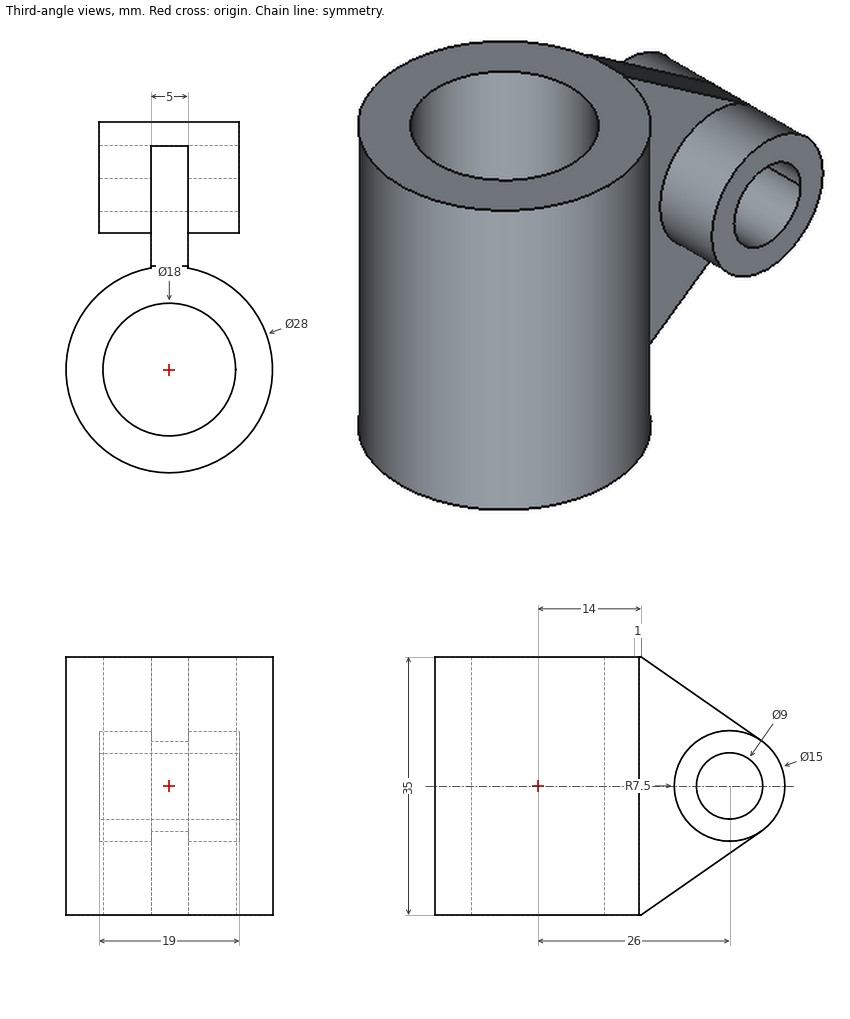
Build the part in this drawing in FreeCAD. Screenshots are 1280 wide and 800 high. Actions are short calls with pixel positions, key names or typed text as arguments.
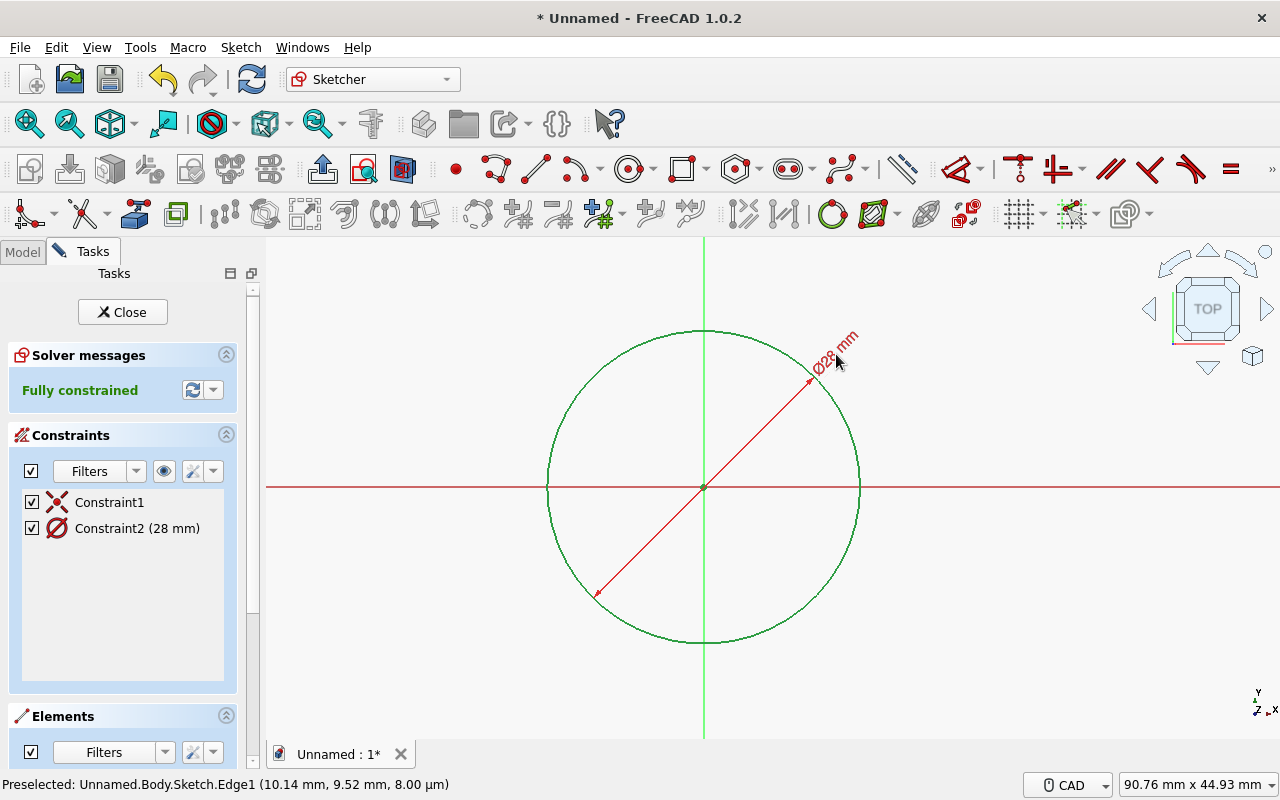
click(123, 312)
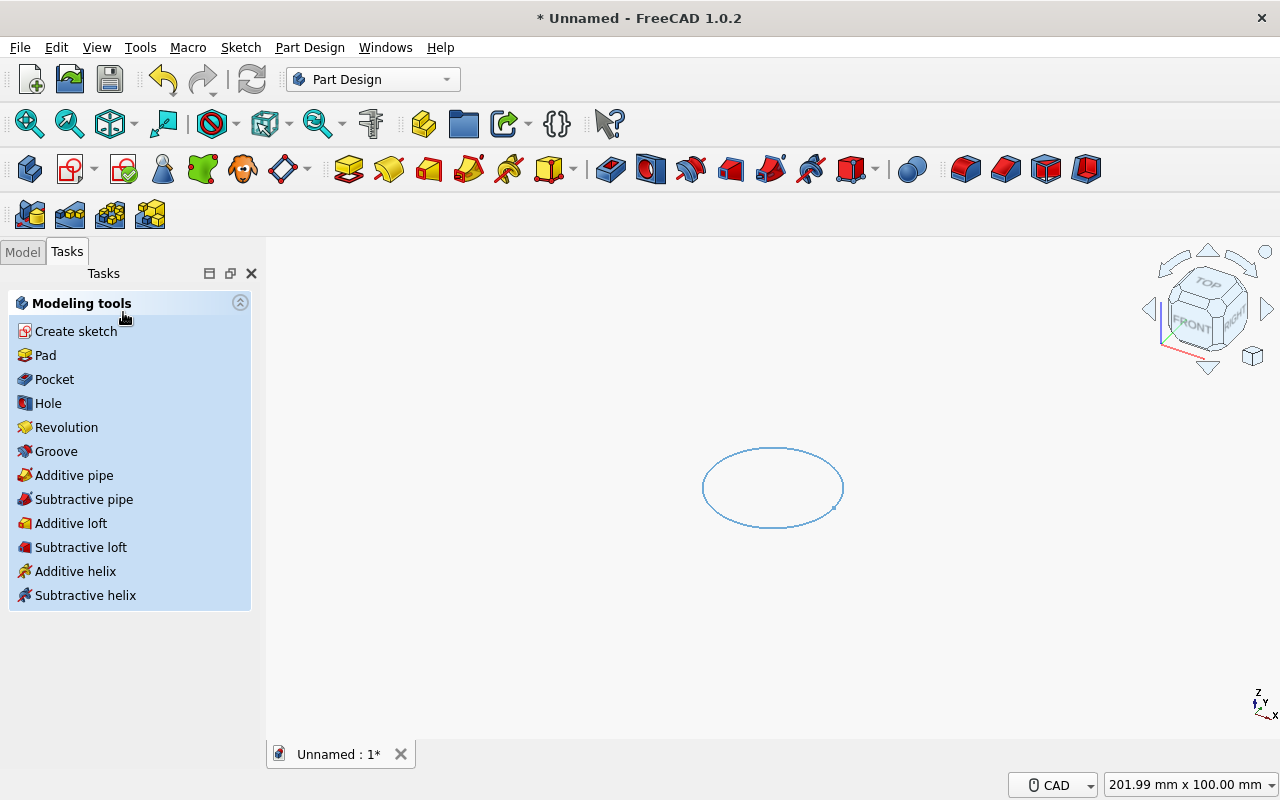
click(350, 170)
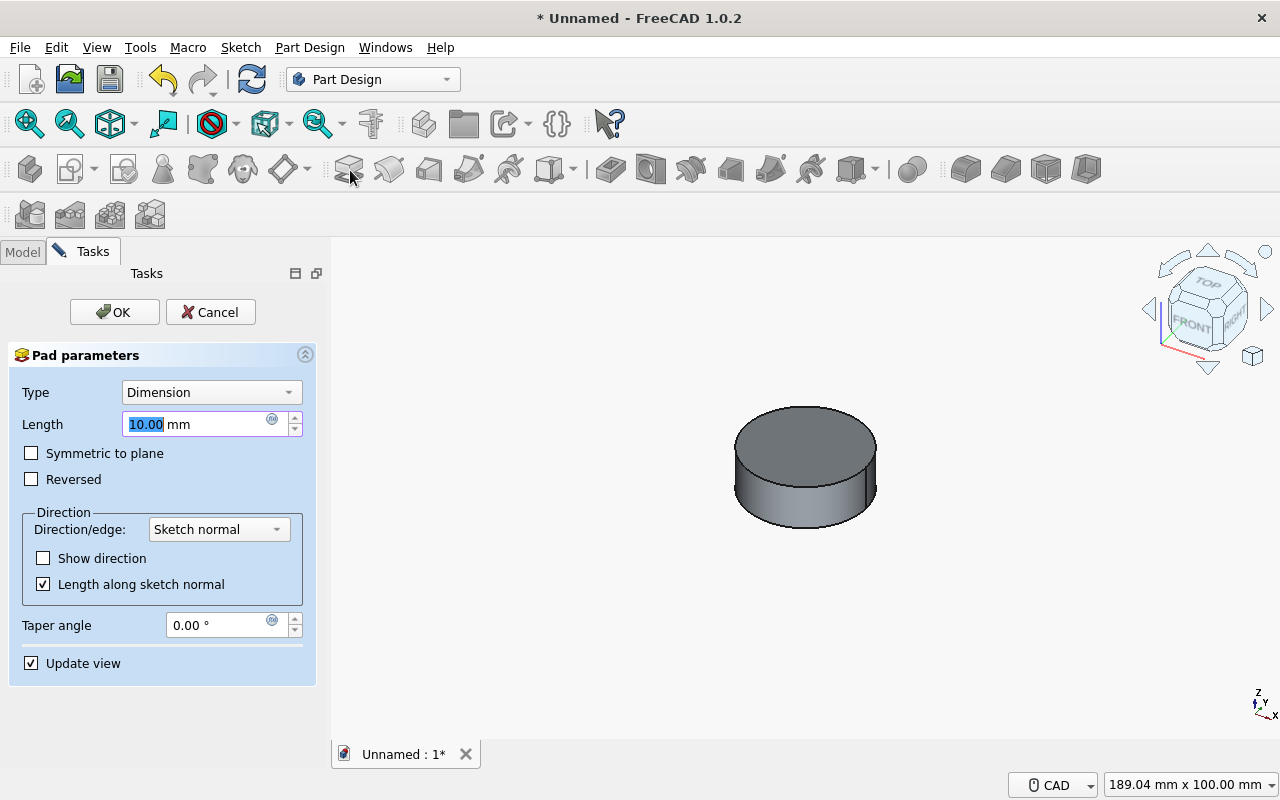
text(35)
key(Tab)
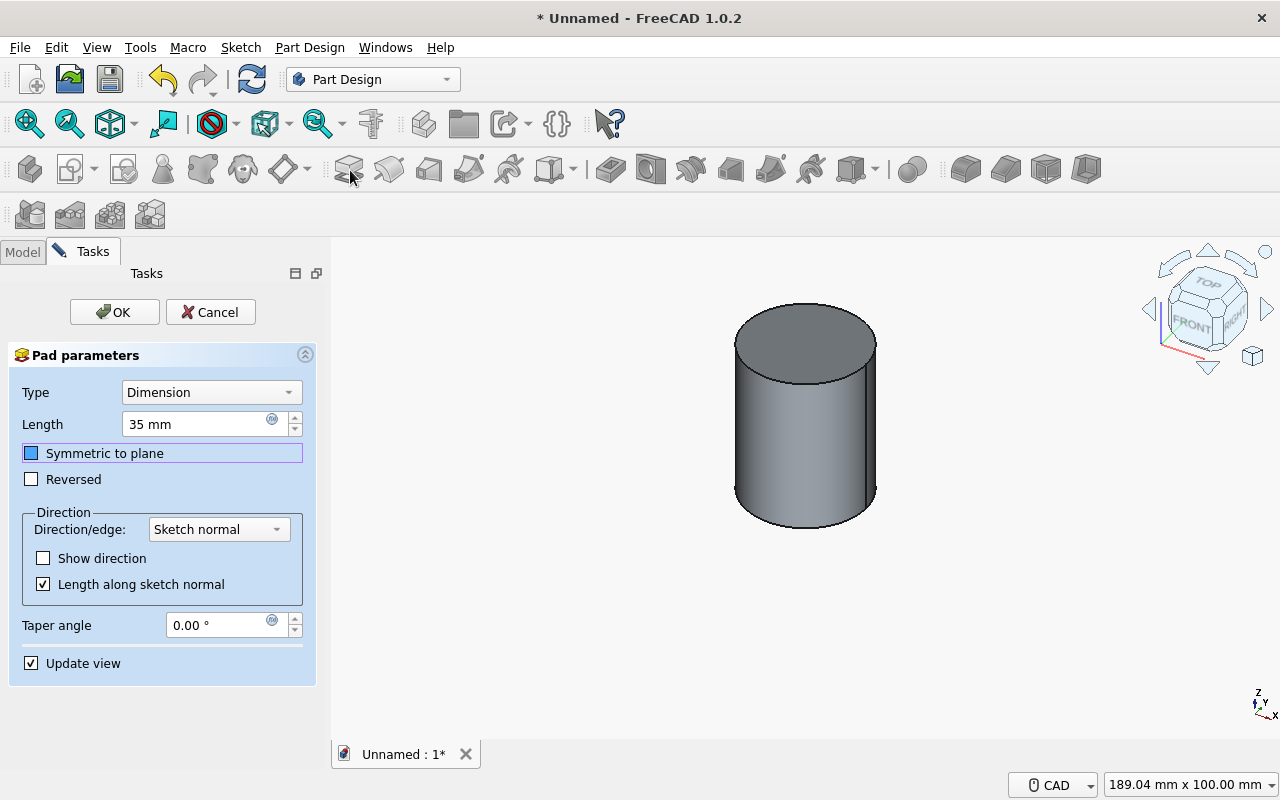
click(30, 453)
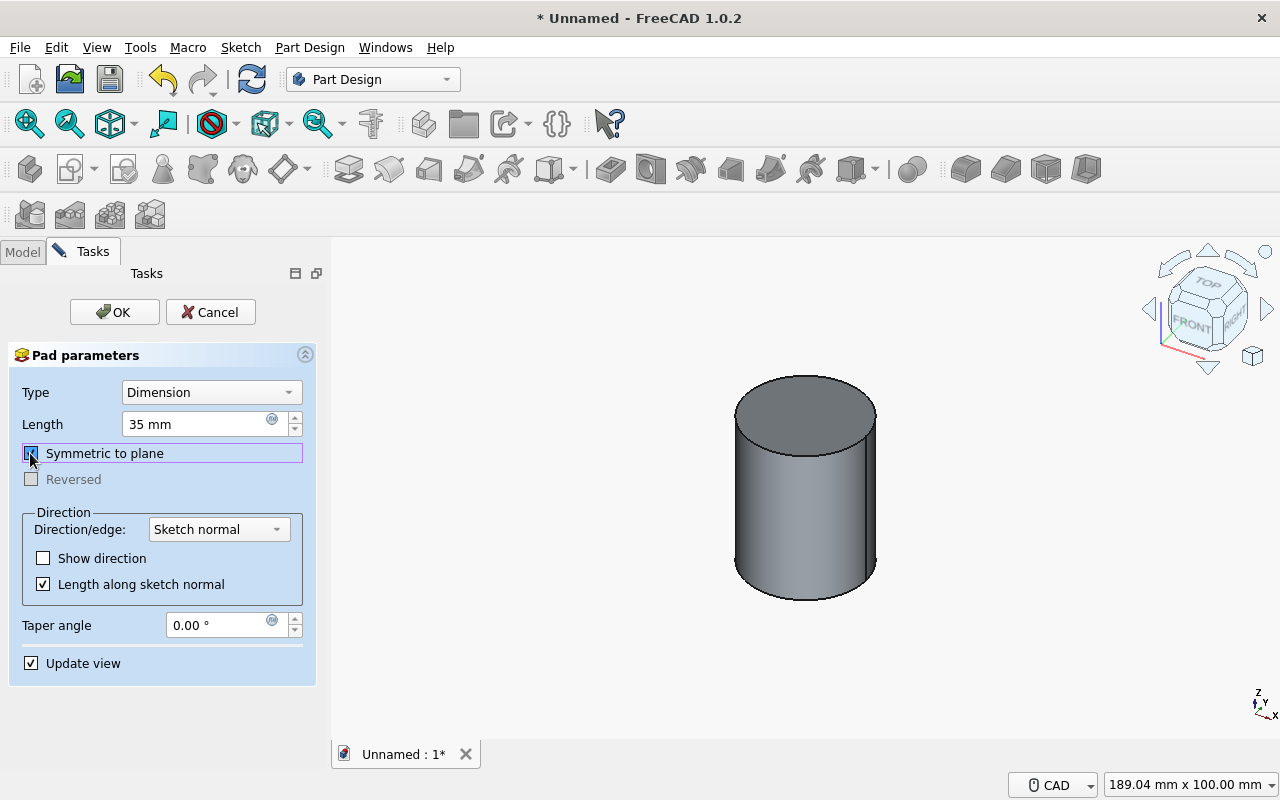
click(115, 312)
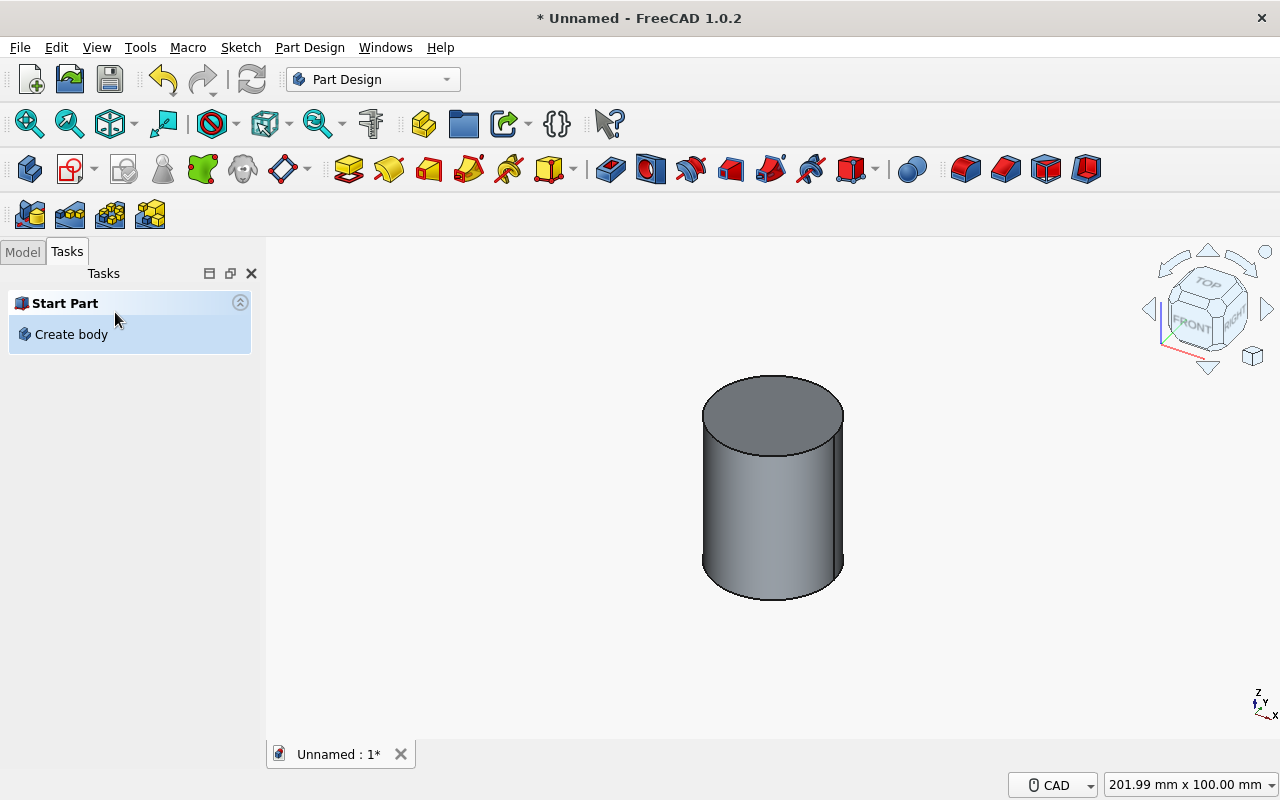
click(773, 415)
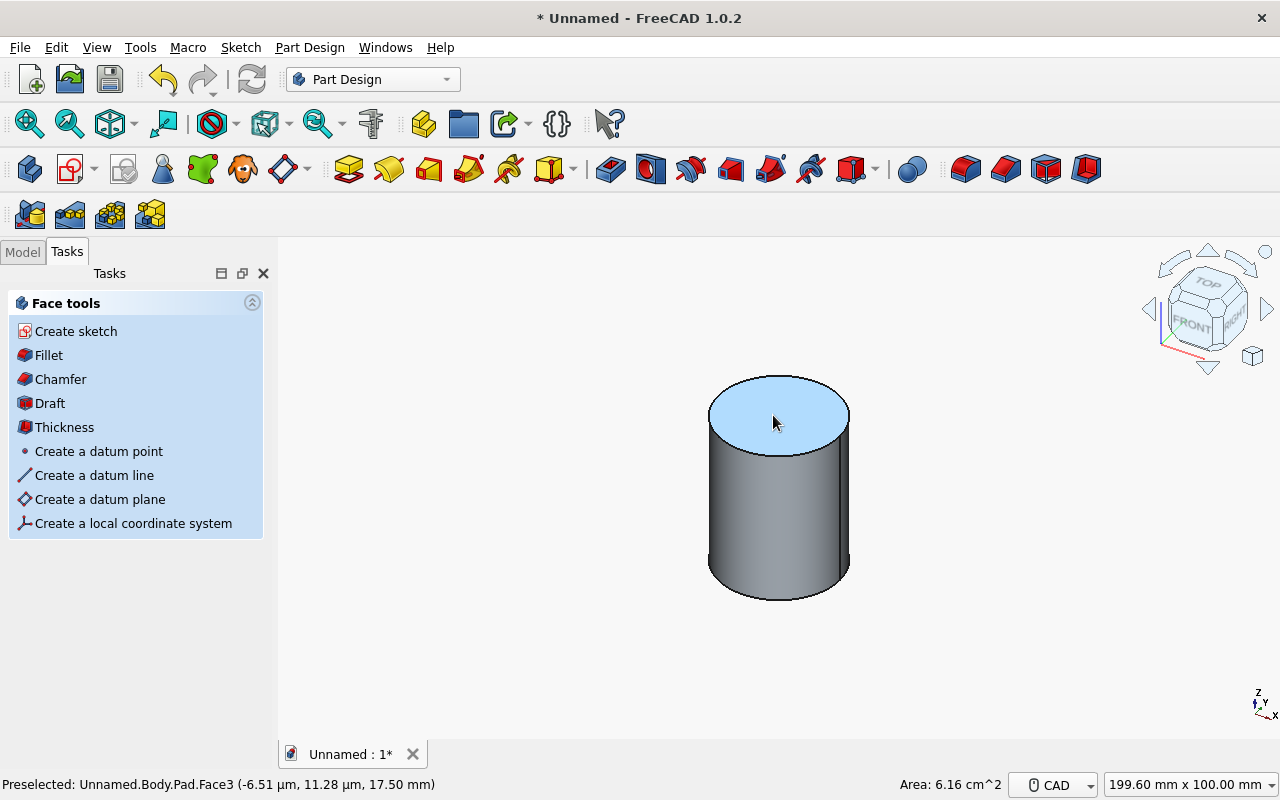
click(70, 170)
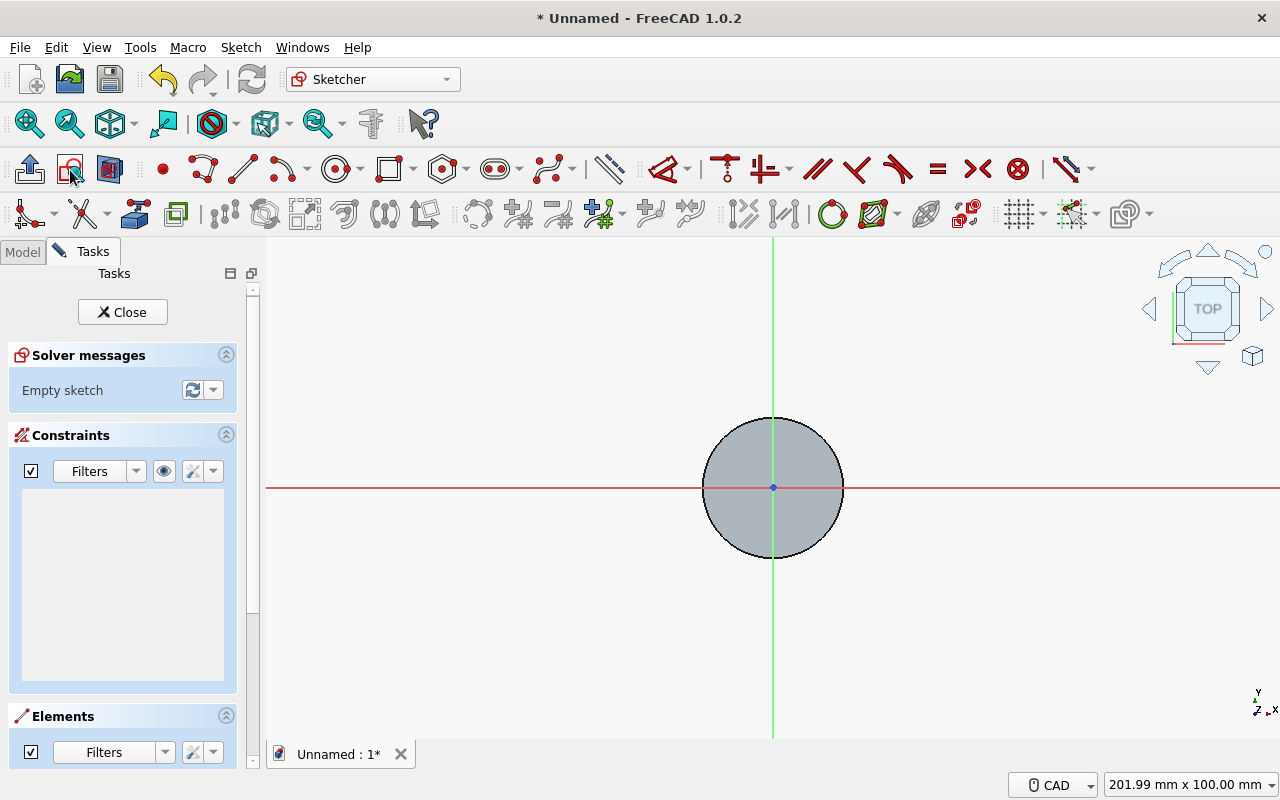
scroll(803, 488, up, 6)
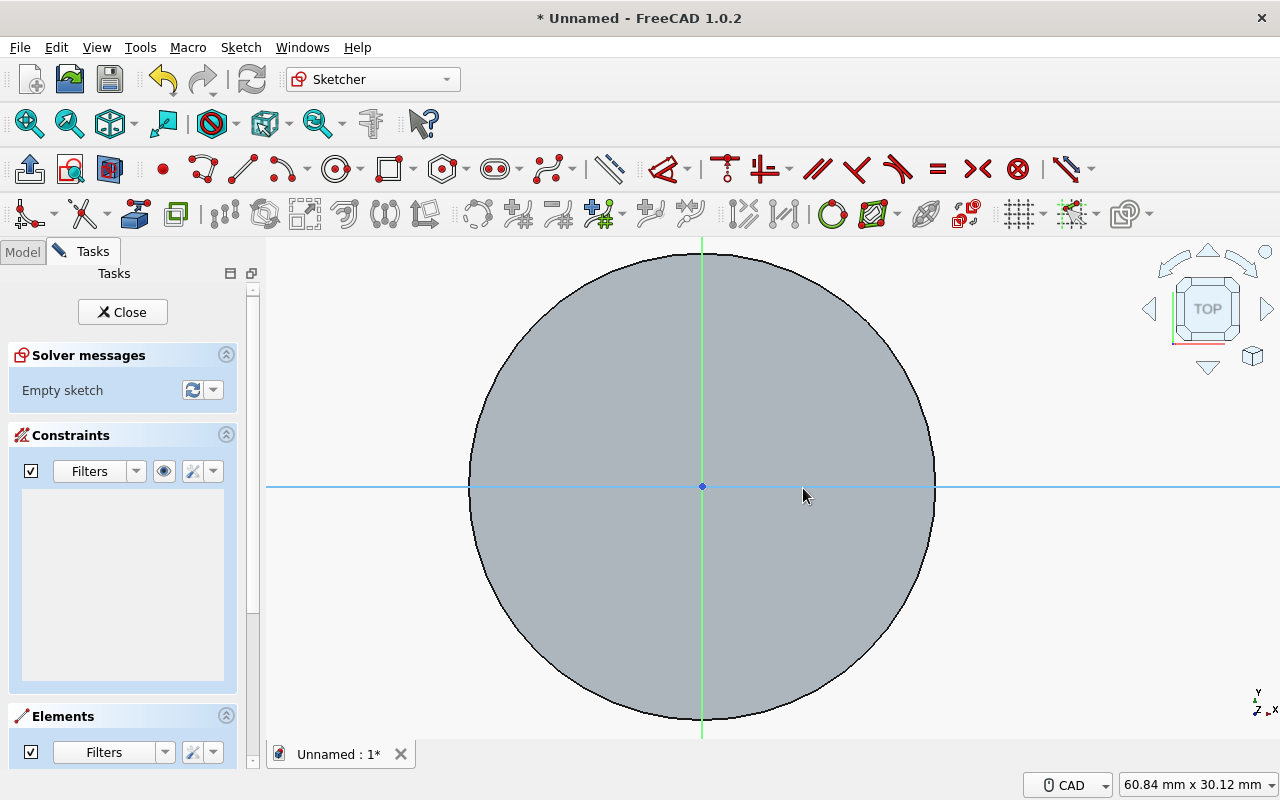
click(336, 170)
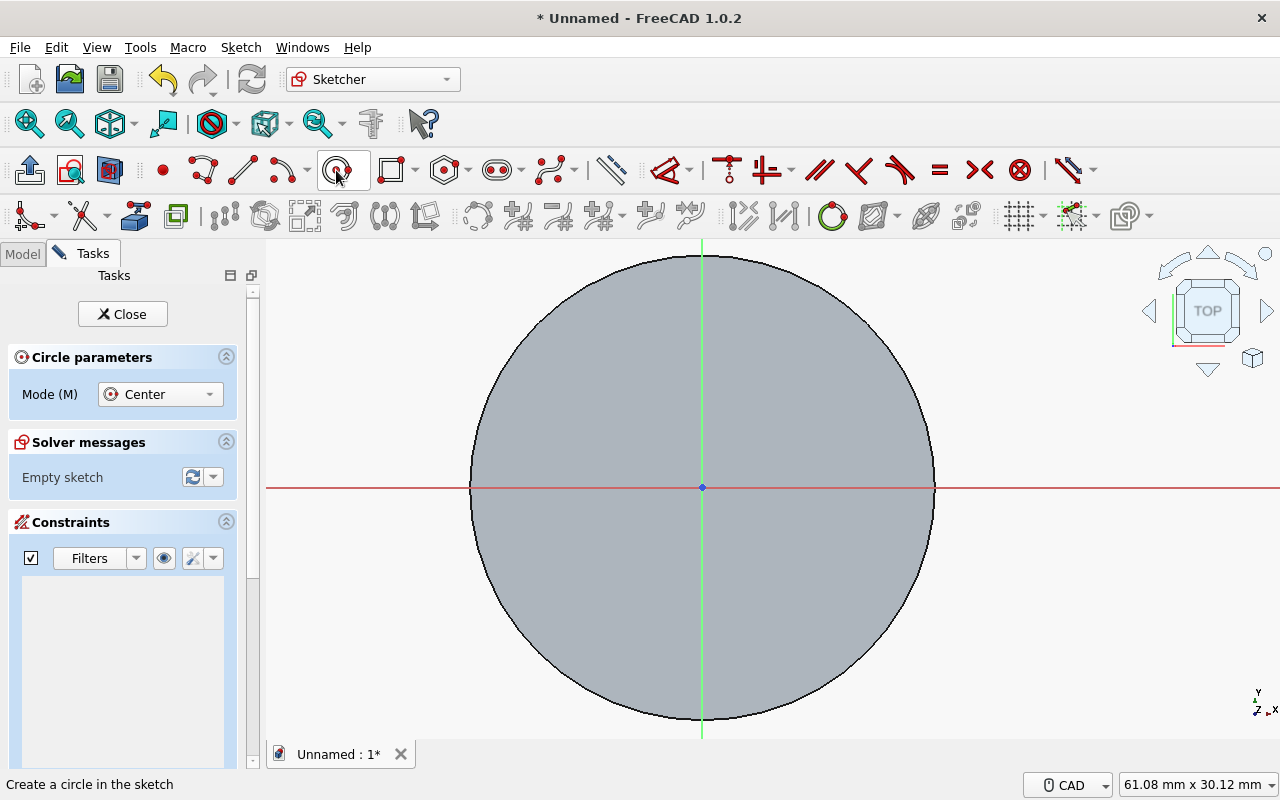
click(702, 488)
click(808, 382)
key(Escape)